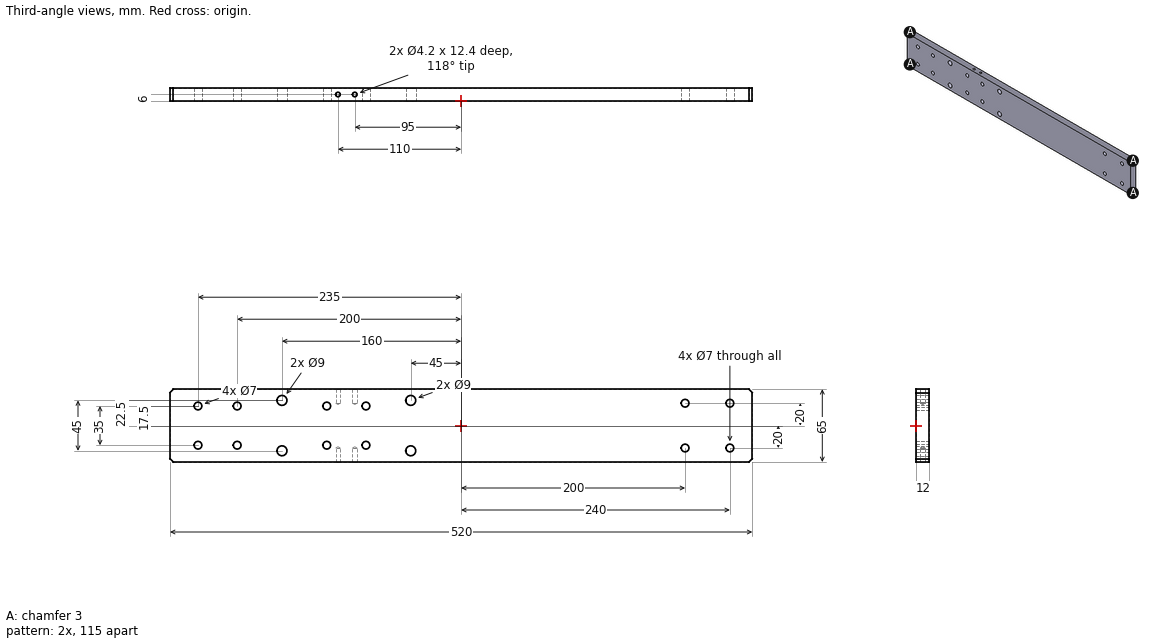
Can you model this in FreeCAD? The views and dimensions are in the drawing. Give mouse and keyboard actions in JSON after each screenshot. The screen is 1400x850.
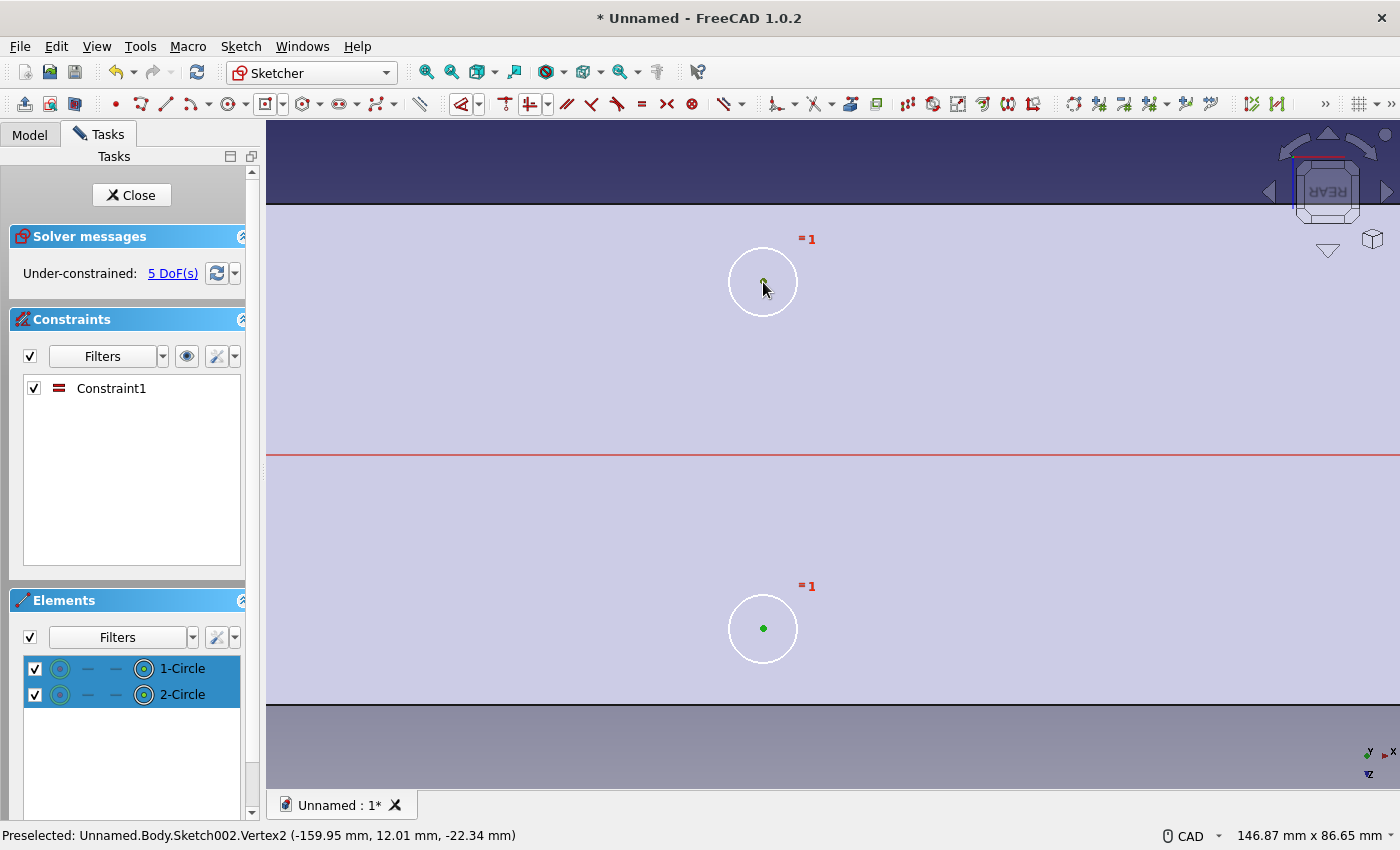
{"action": "left_click", "coordinate": [548, 104]}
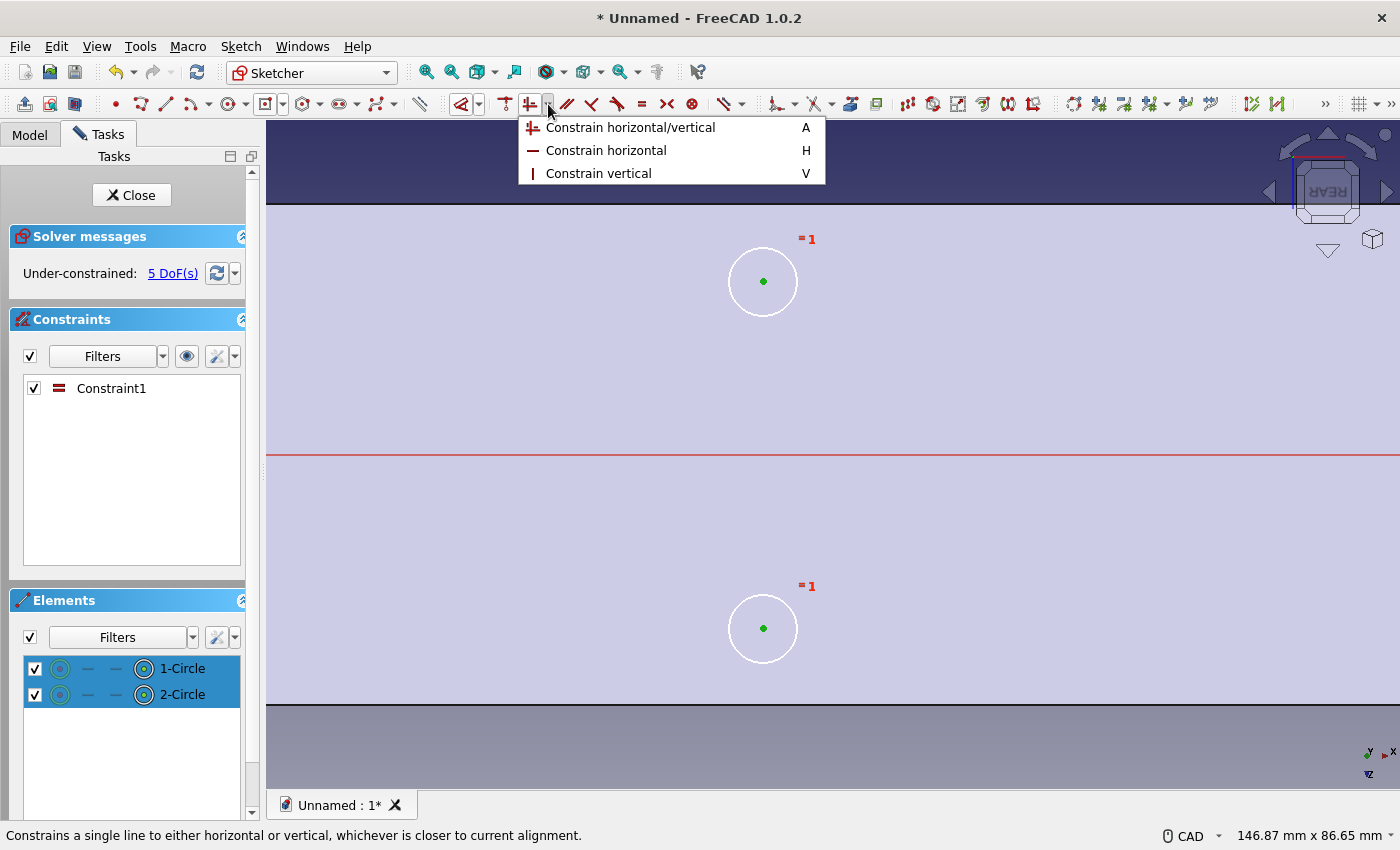
{"action": "left_click", "coordinate": [672, 174]}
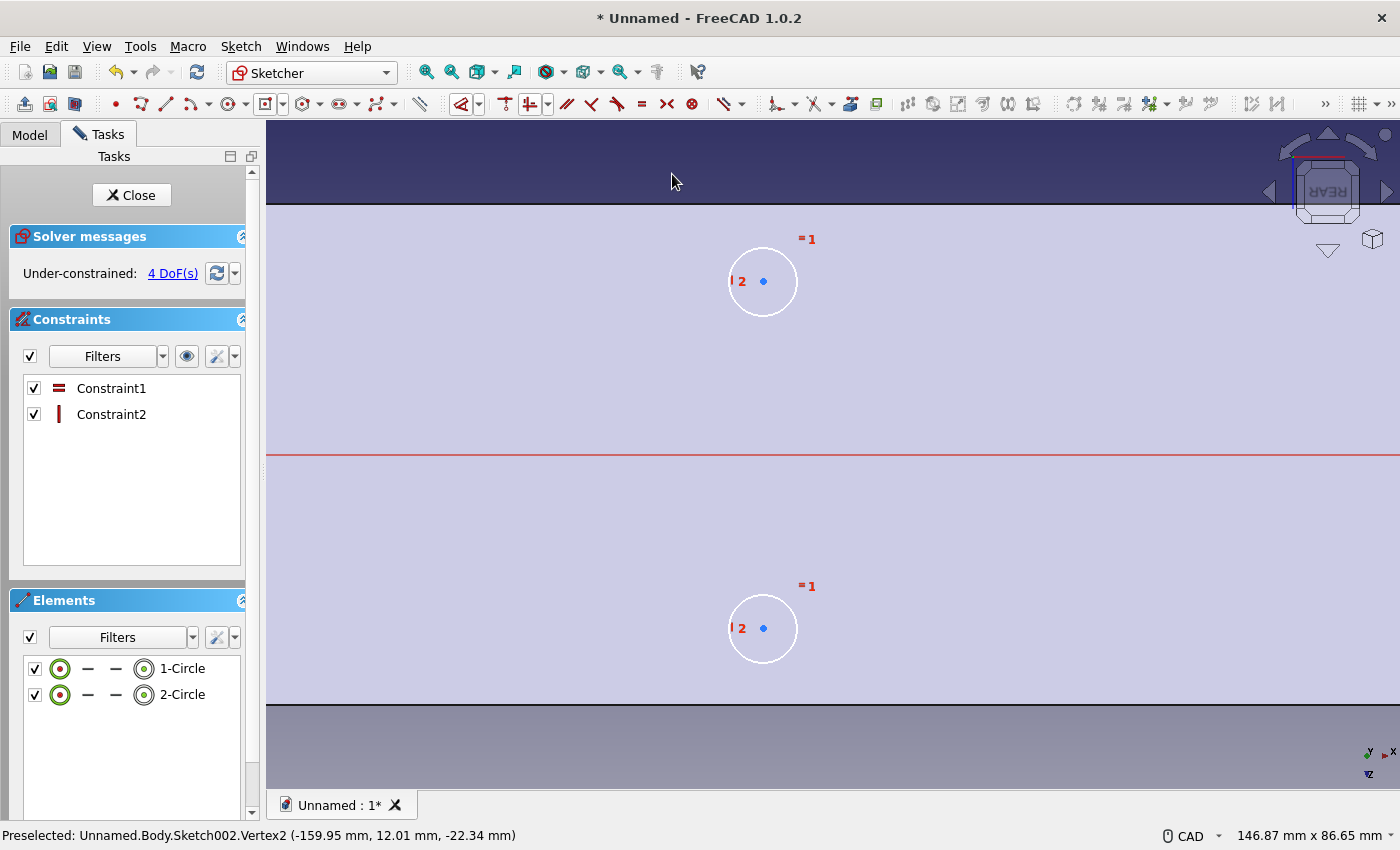
{"action": "left_click", "coordinate": [787, 605]}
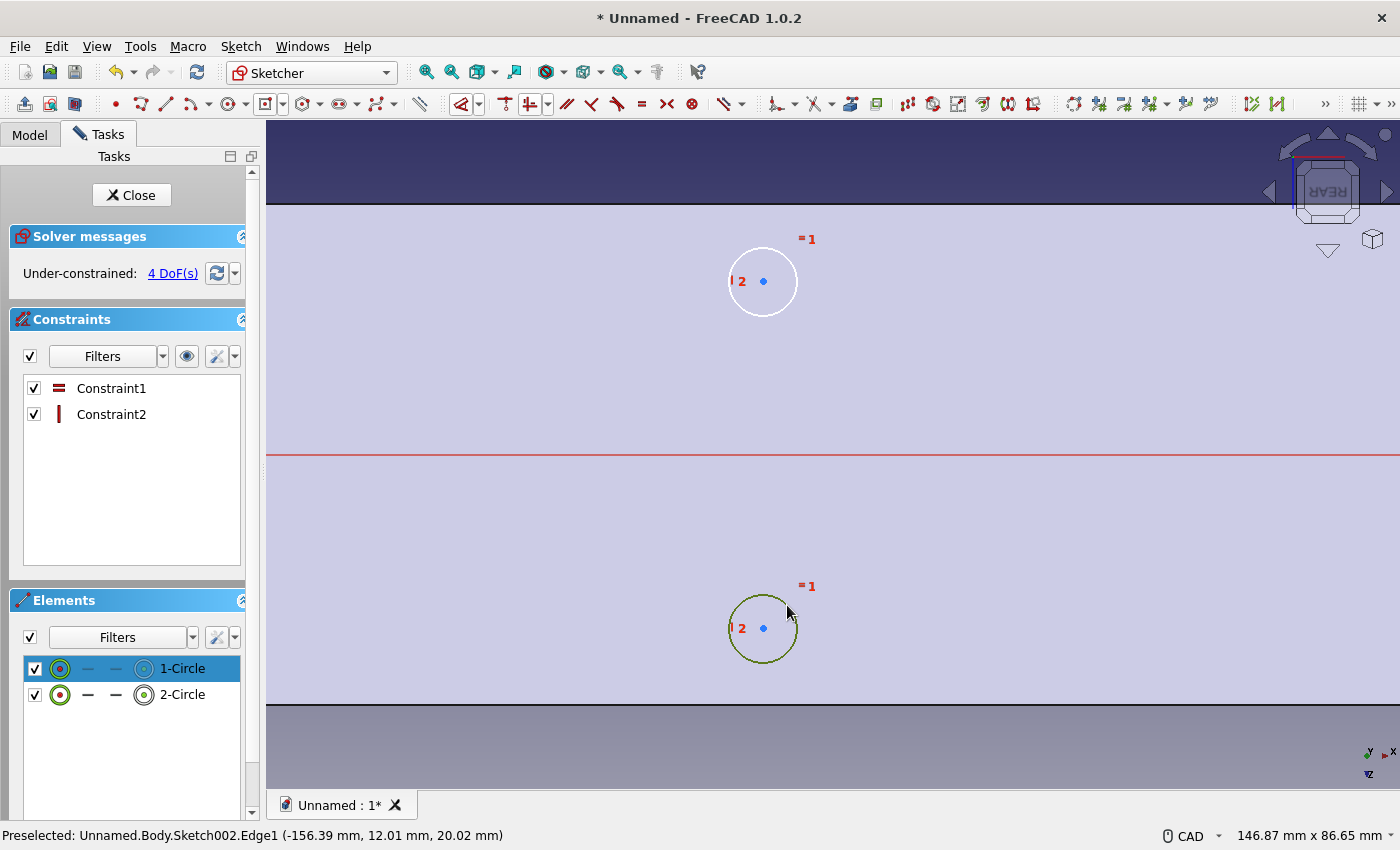
{"action": "left_click", "coordinate": [478, 104]}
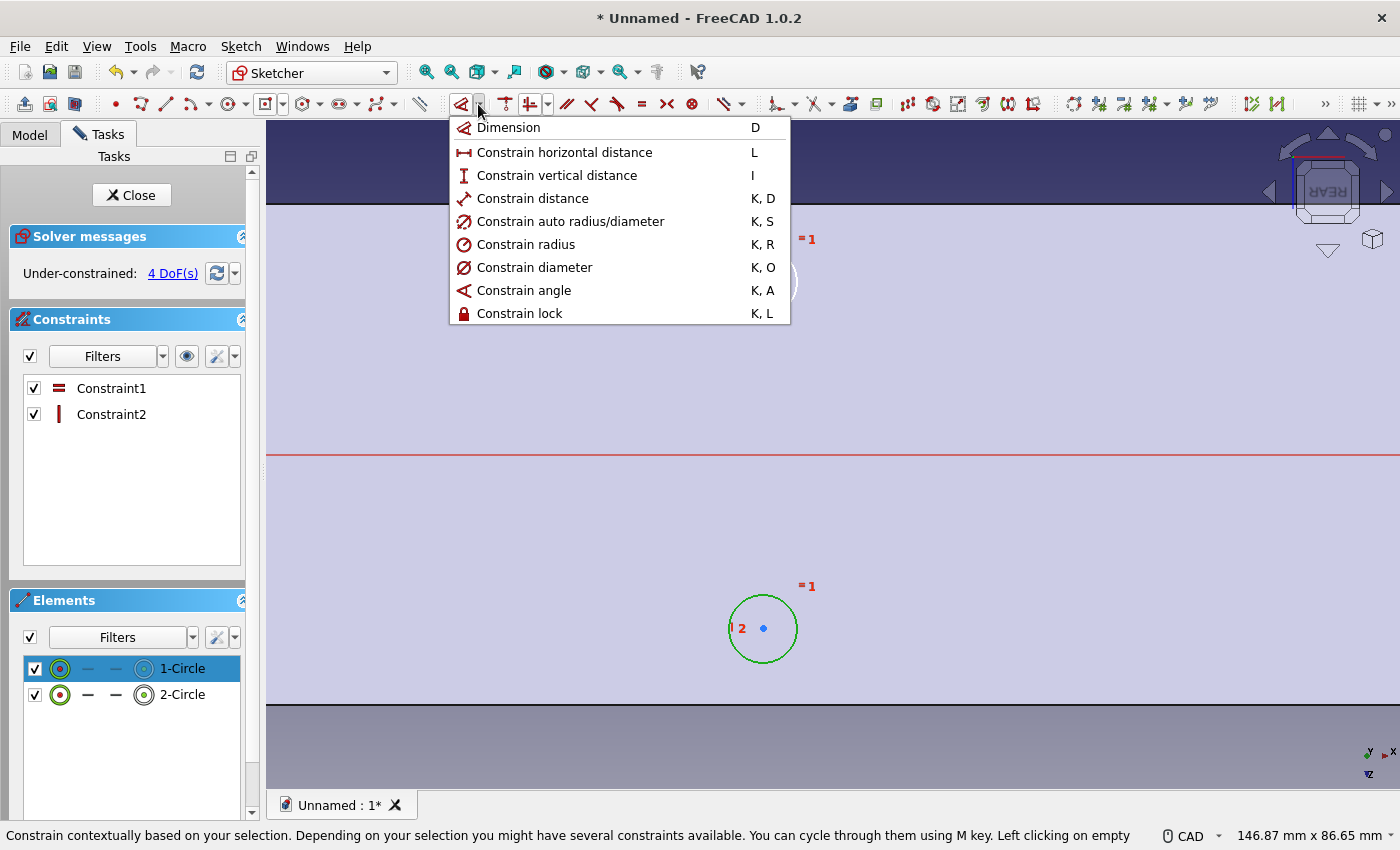
{"action": "left_click", "coordinate": [620, 268]}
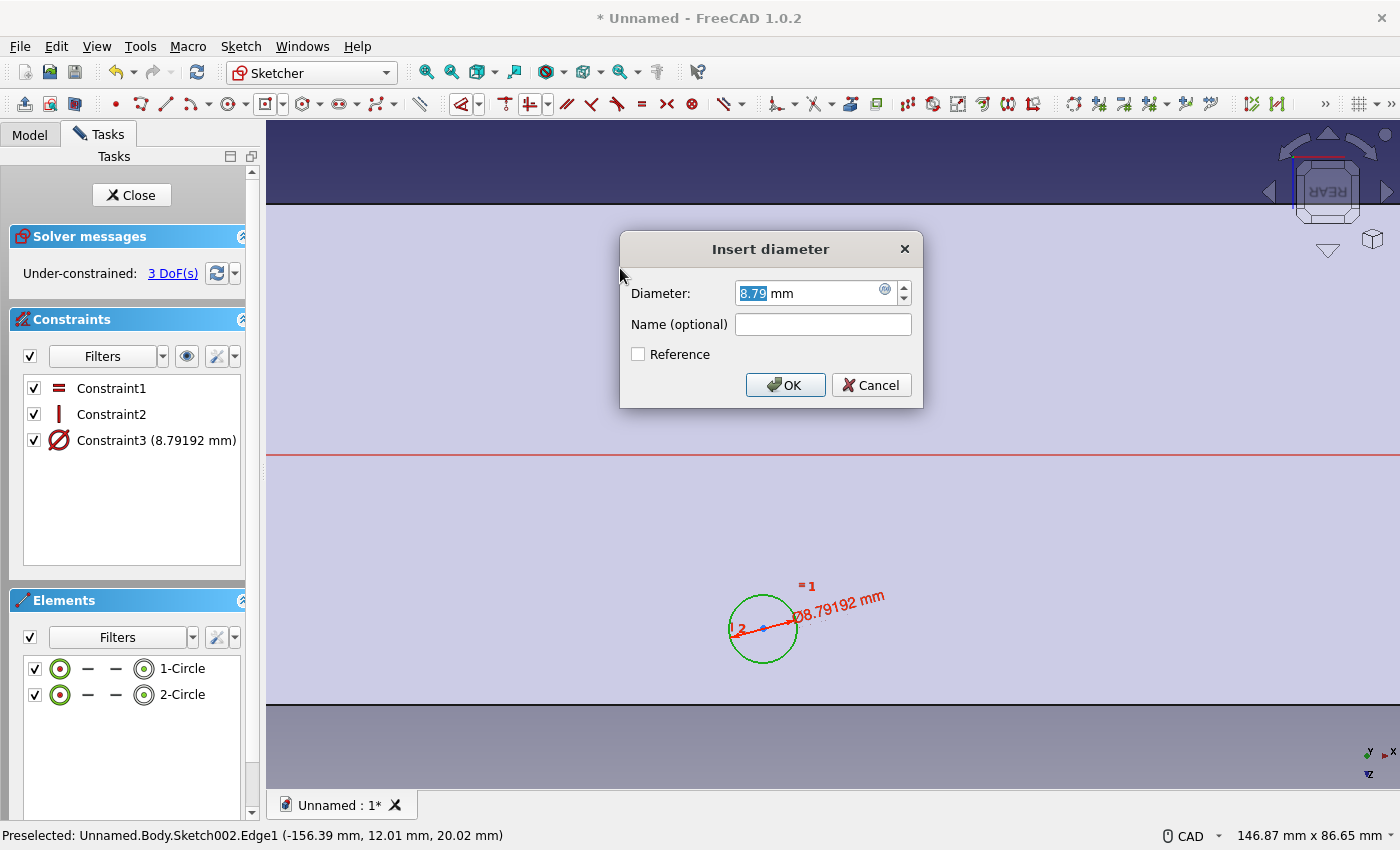
{"action": "type", "text": "9"}
{"action": "key", "text": "Return"}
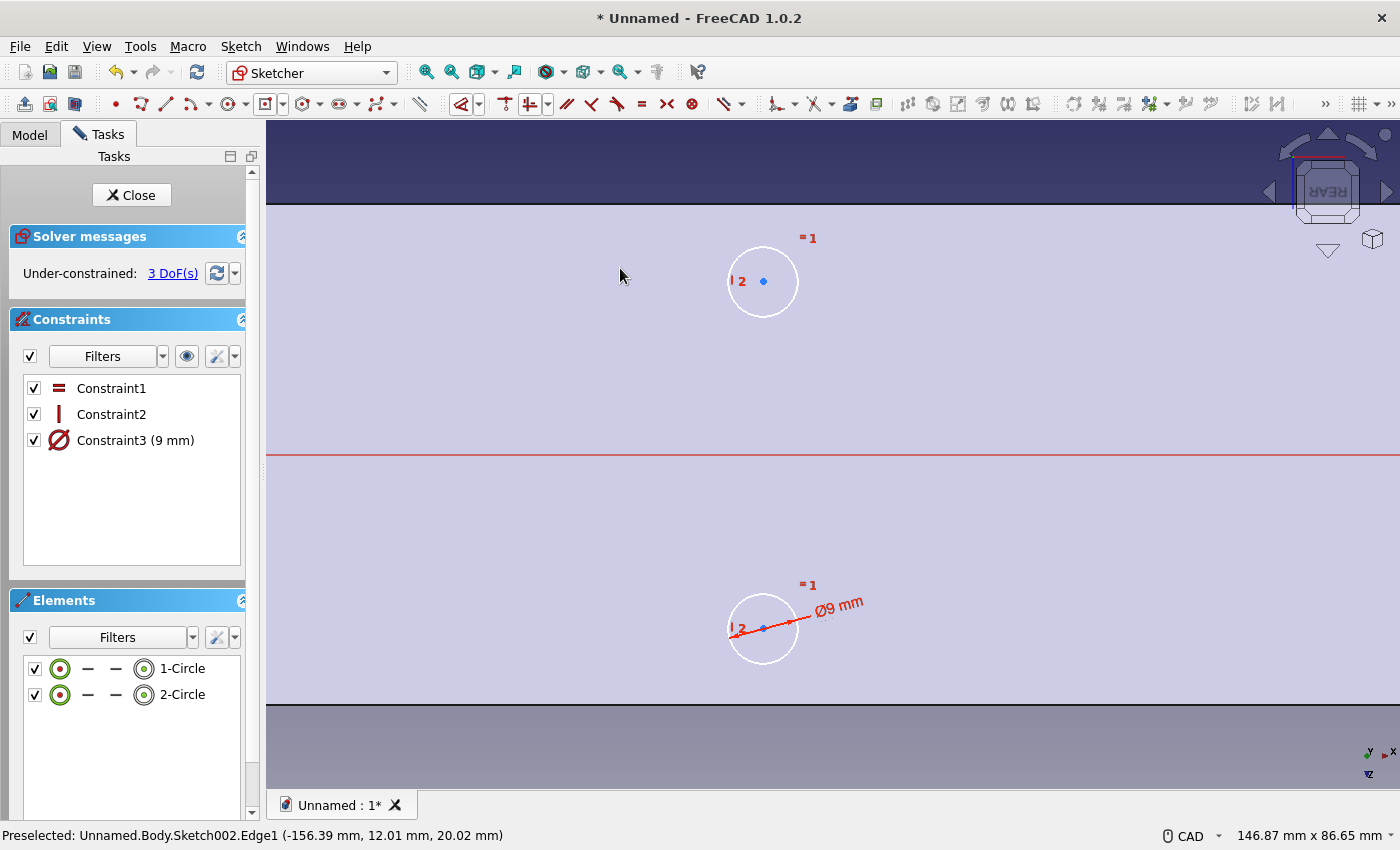
{"action": "left_click", "coordinate": [763, 629]}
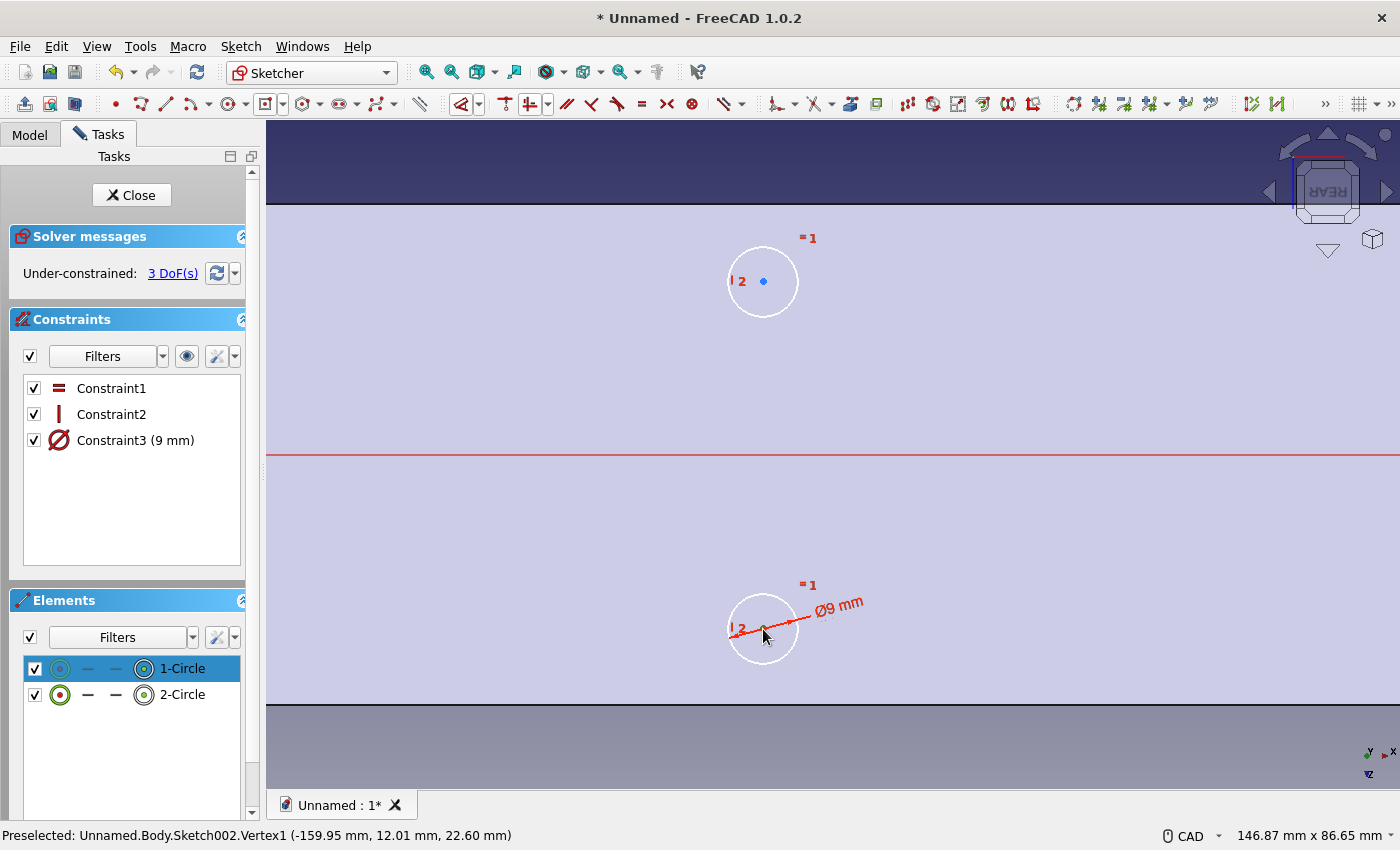
{"action": "key", "text": "l"}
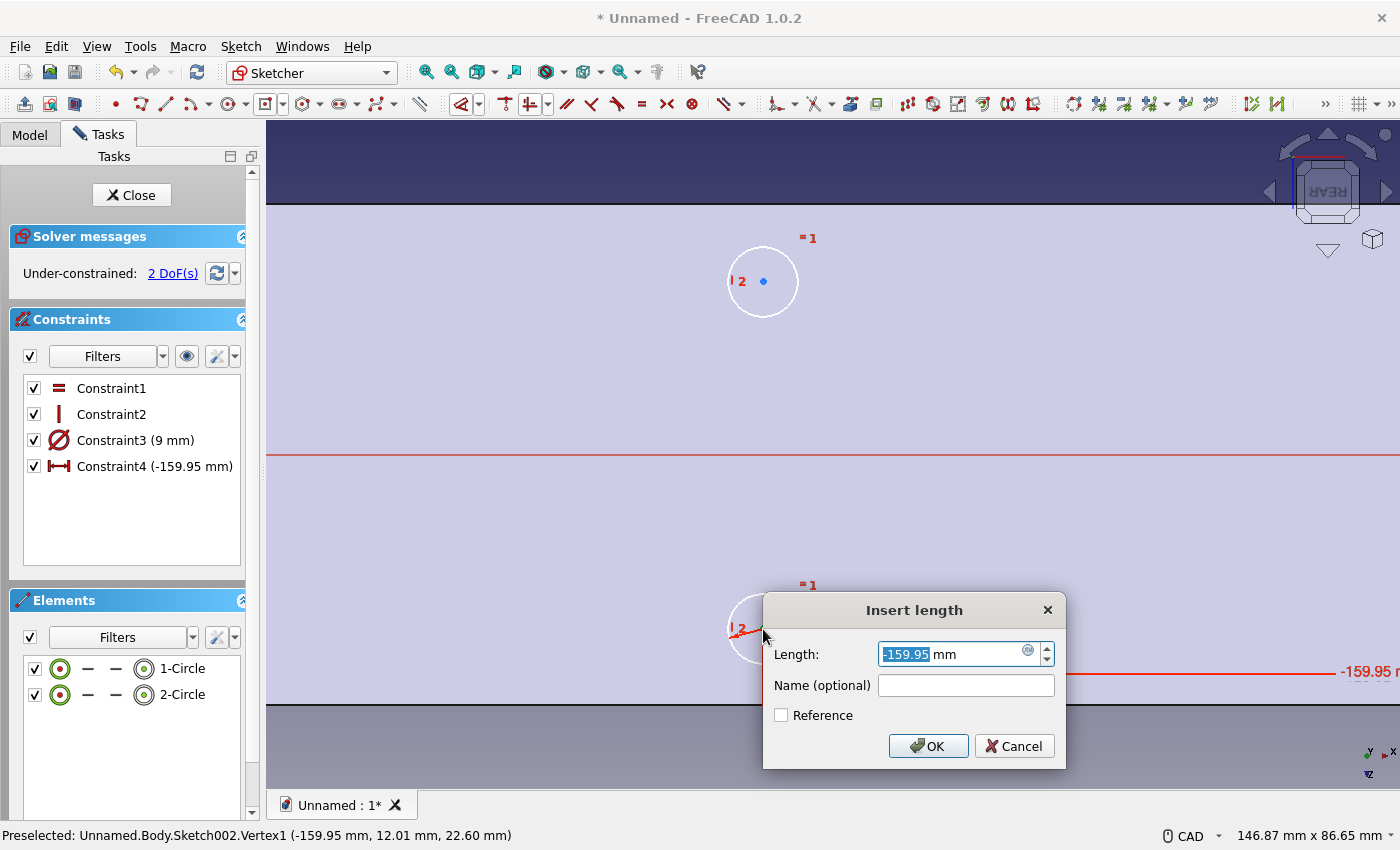
{"action": "type", "text": "-160"}
{"action": "key", "text": "Return"}